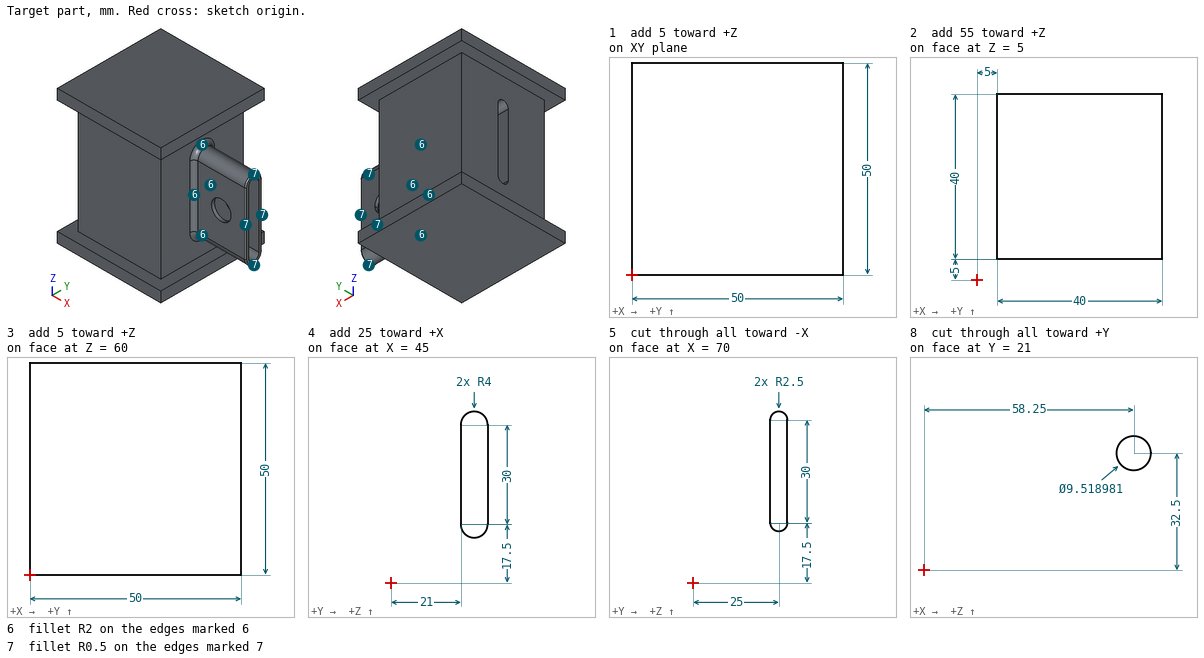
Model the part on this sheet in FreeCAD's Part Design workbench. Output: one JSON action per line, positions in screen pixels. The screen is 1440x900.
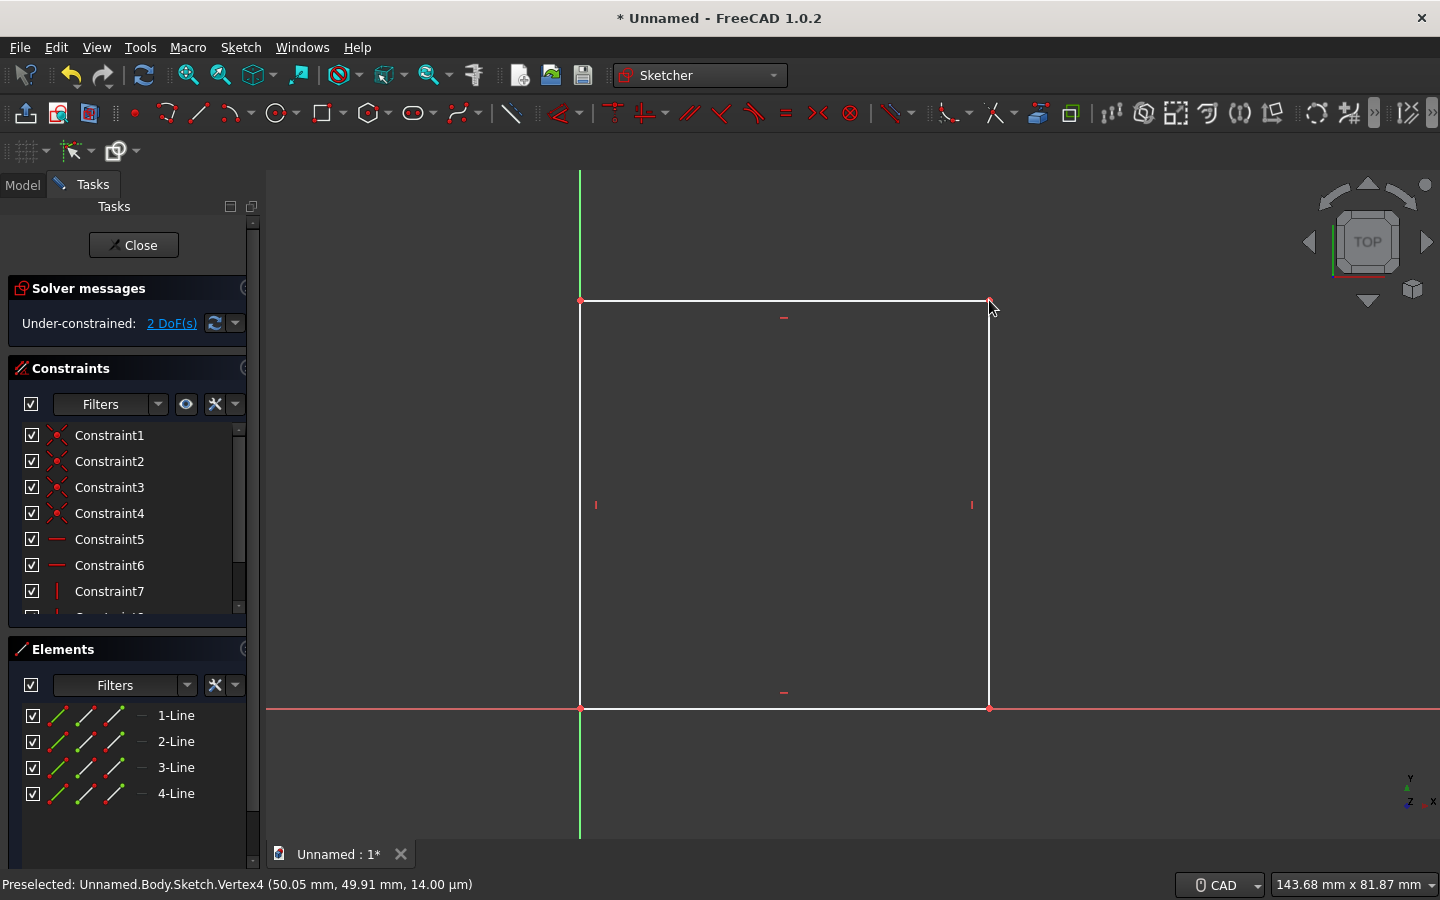
{"action": "left_click", "coordinate": [558, 114]}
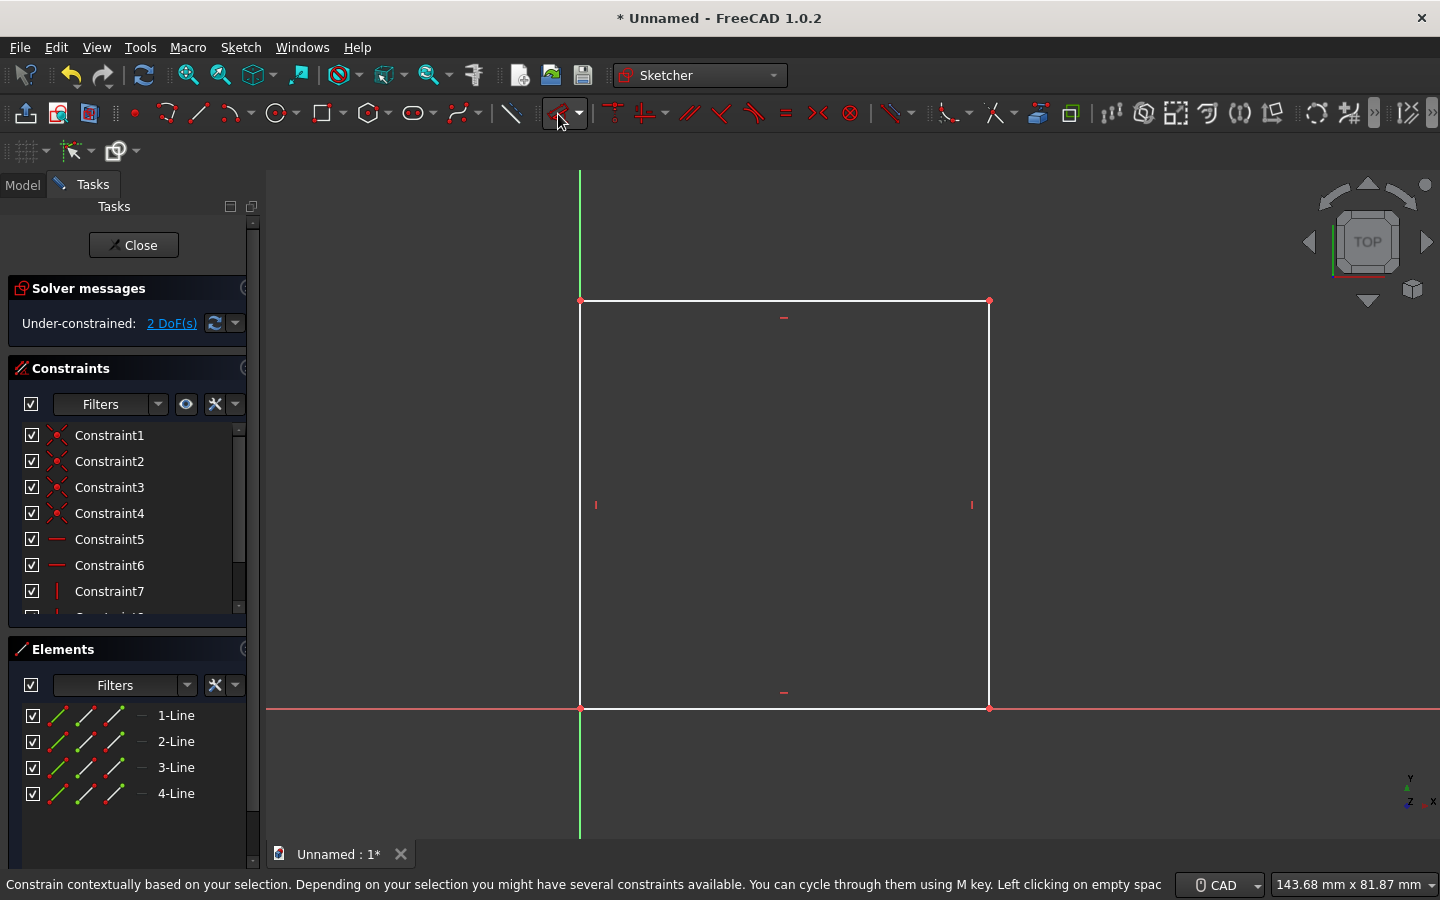
{"action": "left_click", "coordinate": [703, 709]}
{"action": "left_click", "coordinate": [785, 743]}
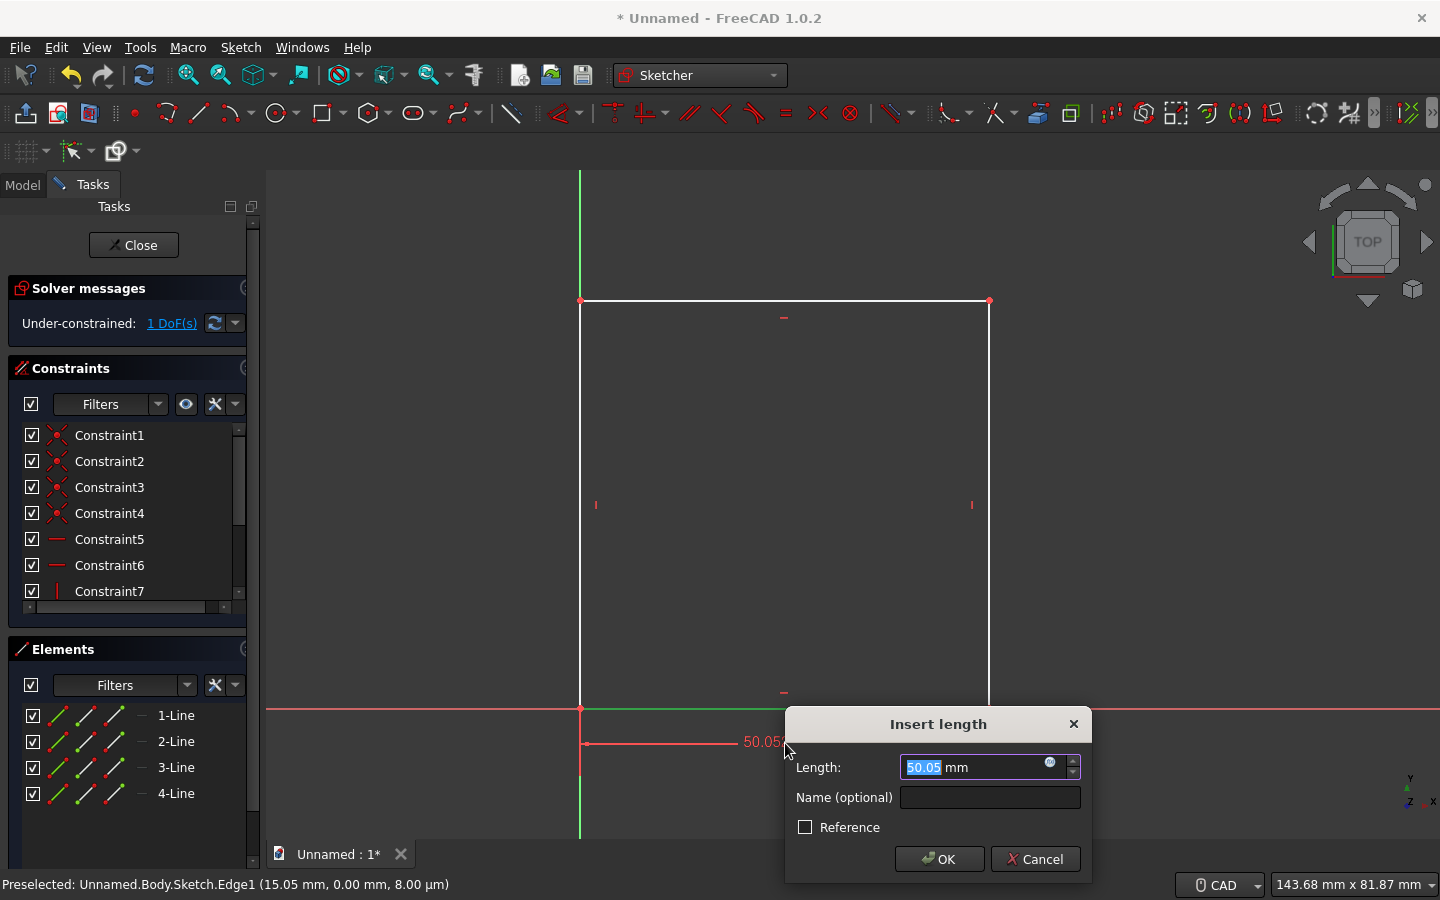
{"action": "type", "text": "50"}
{"action": "key", "text": "Return"}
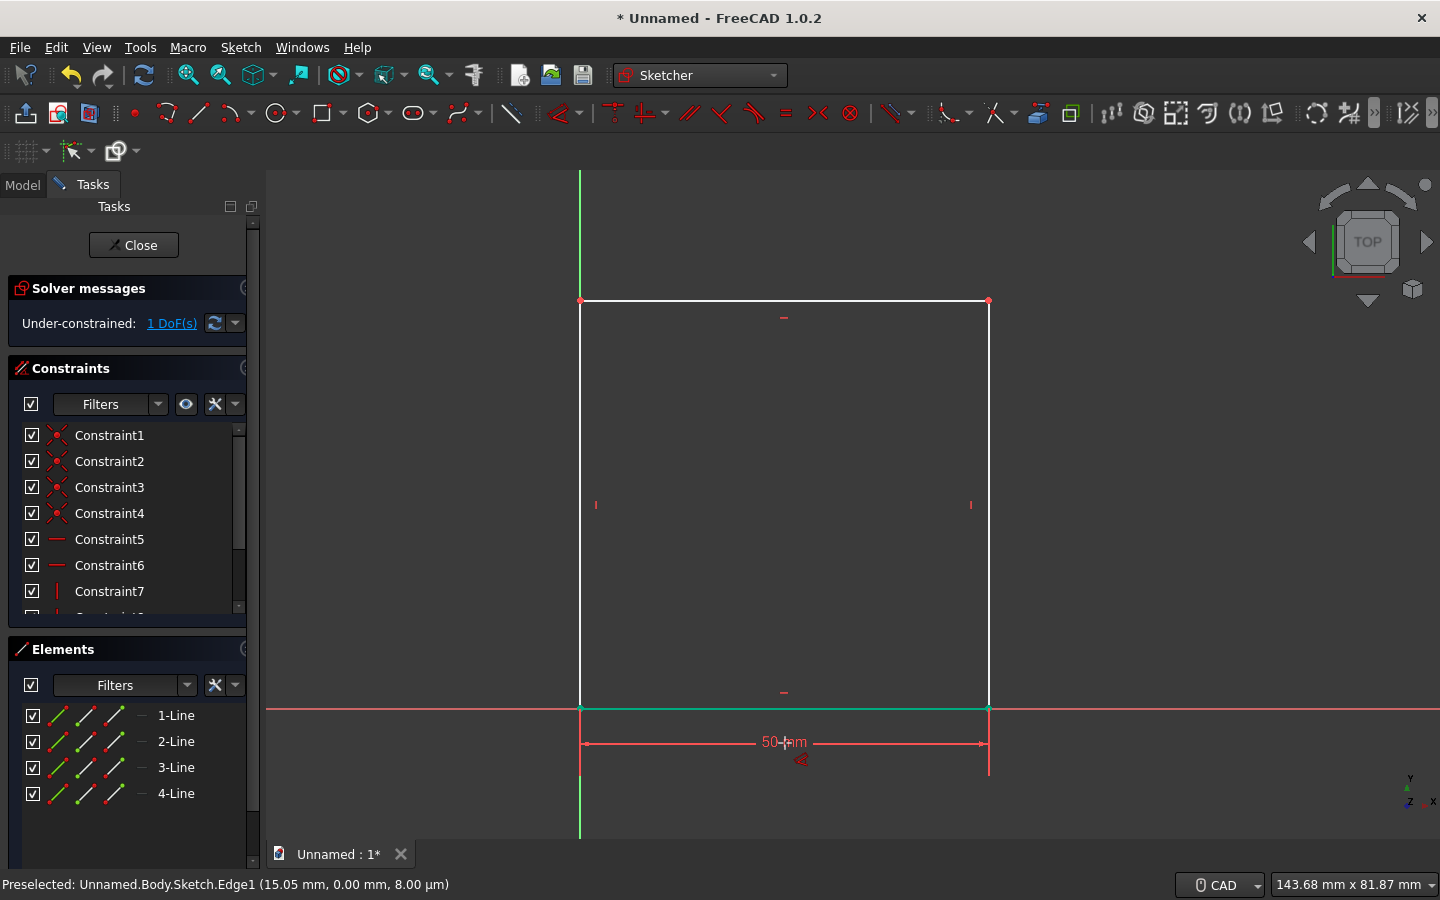
{"action": "left_click", "coordinate": [989, 586]}
{"action": "left_click", "coordinate": [1023, 505]}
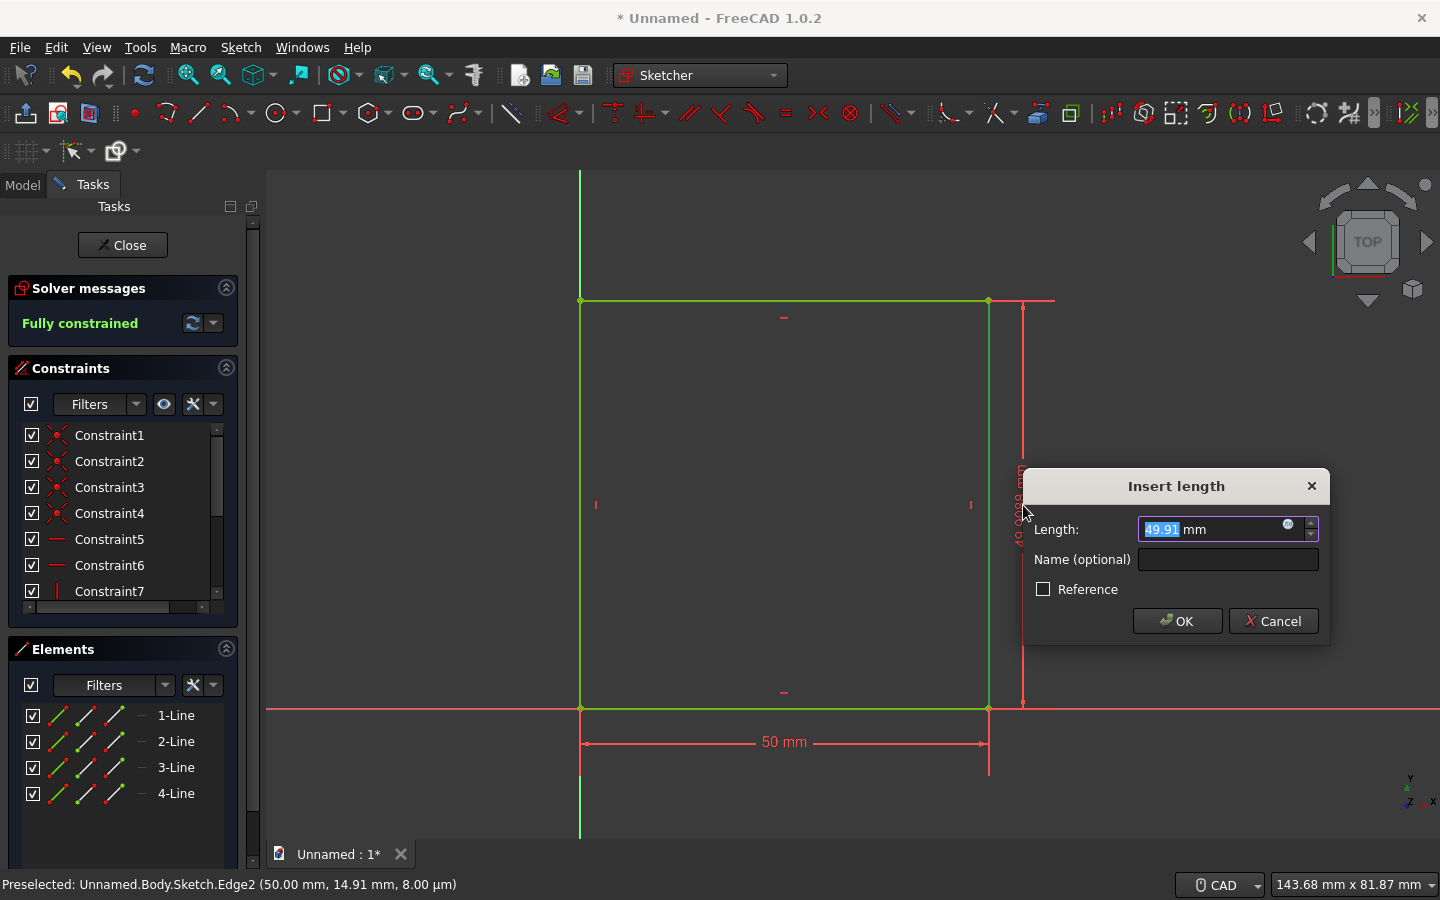
{"action": "type", "text": "50"}
{"action": "key", "text": "Return"}
{"action": "key", "text": "Escape"}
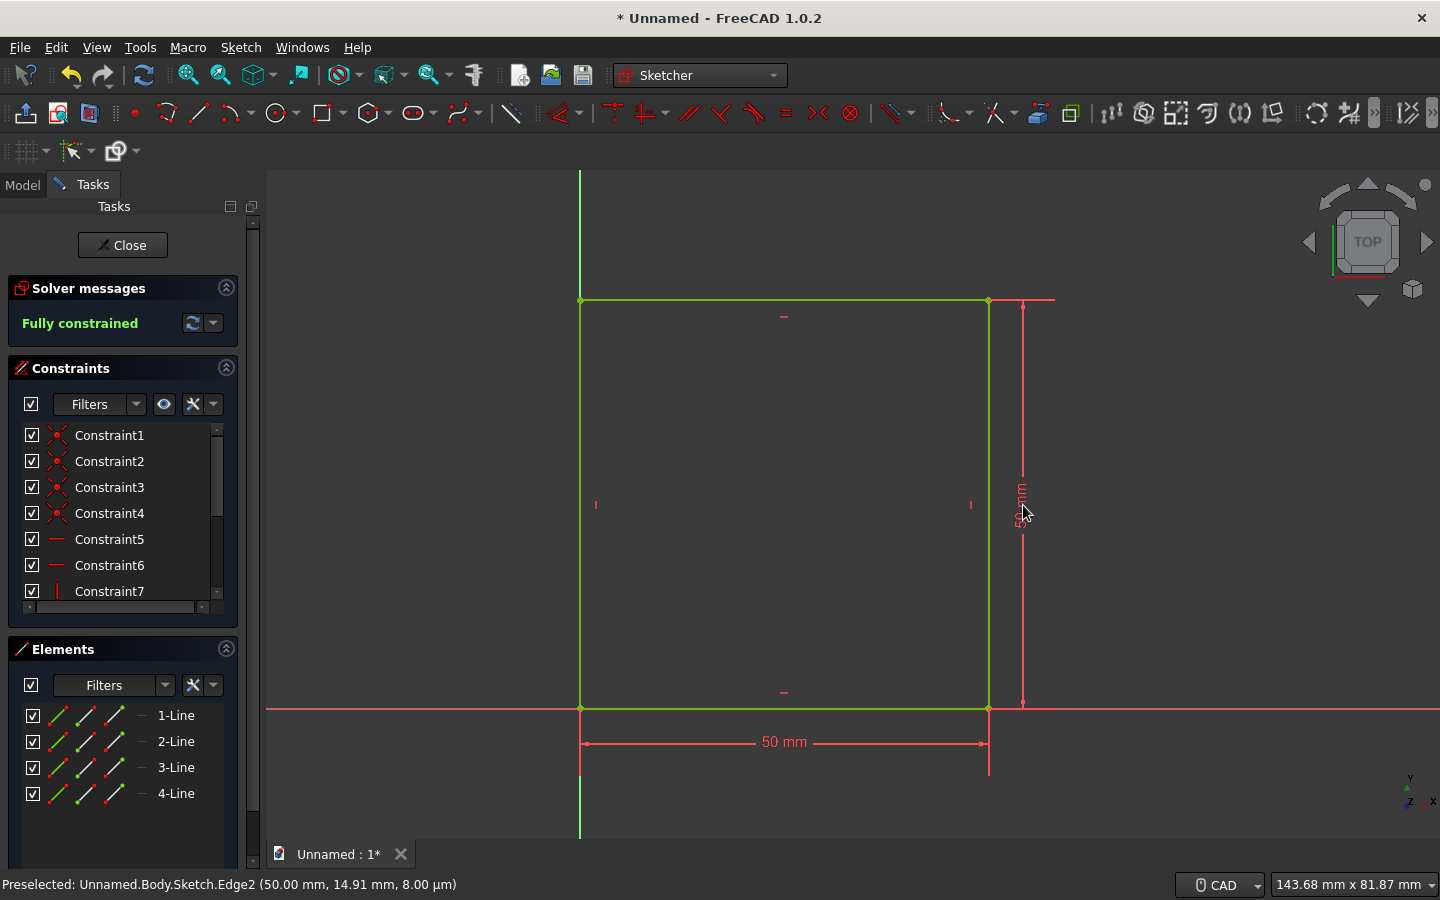
{"action": "left_click", "coordinate": [123, 245]}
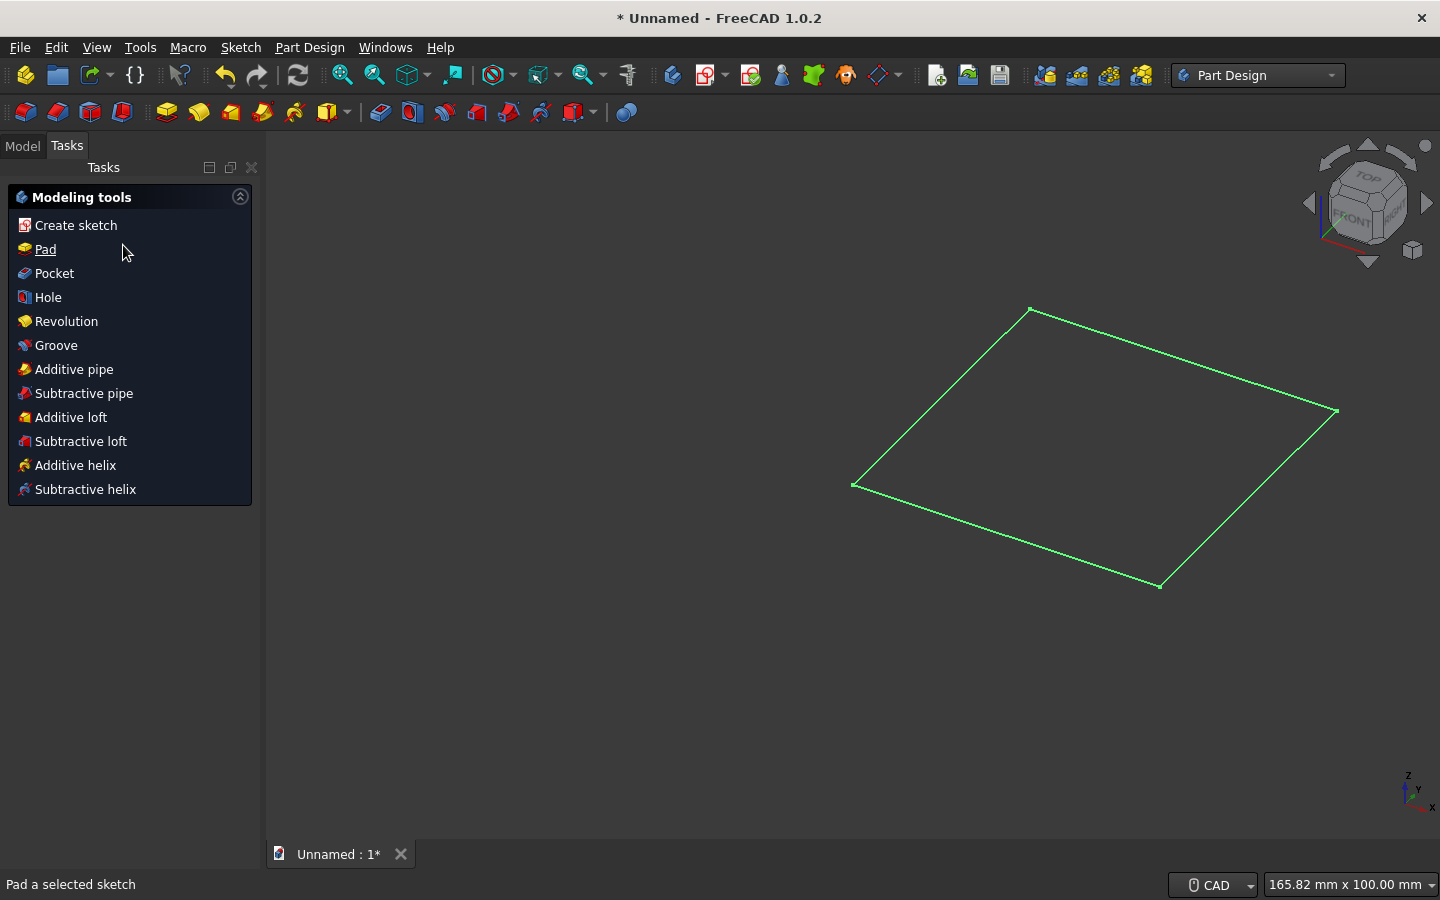
{"action": "left_click", "coordinate": [168, 112]}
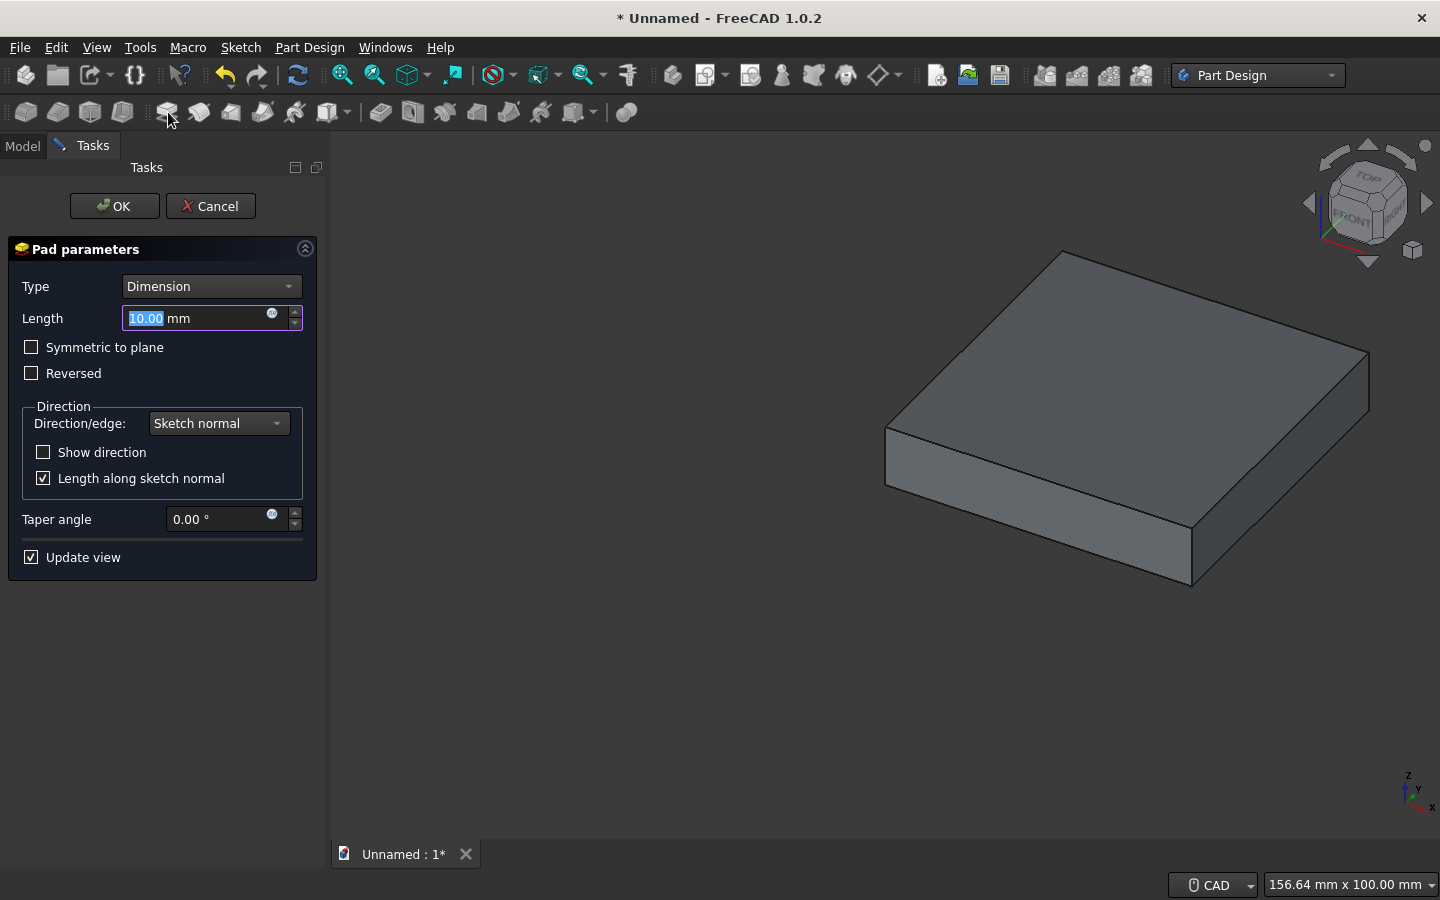
{"action": "type", "text": "5"}
{"action": "key", "text": "Tab"}